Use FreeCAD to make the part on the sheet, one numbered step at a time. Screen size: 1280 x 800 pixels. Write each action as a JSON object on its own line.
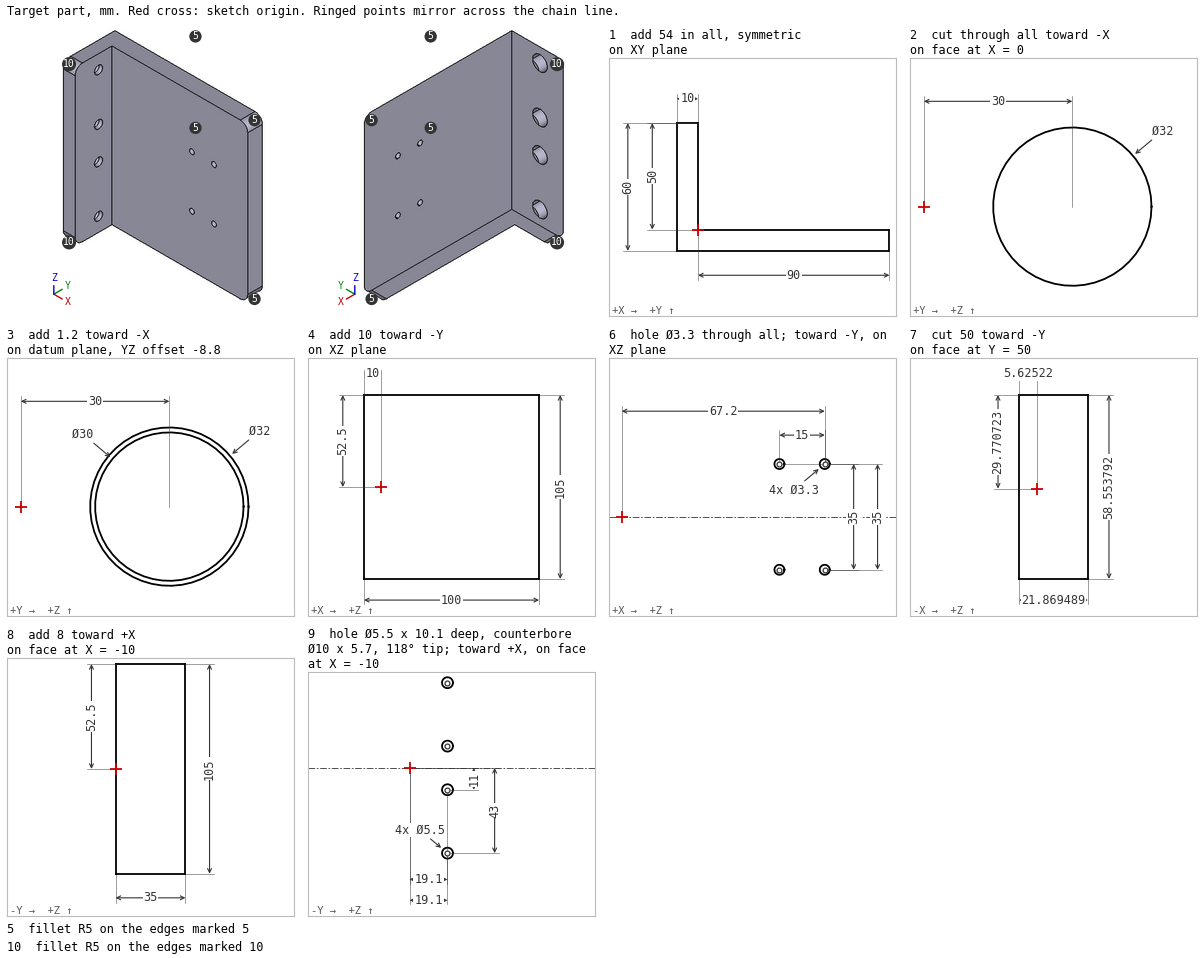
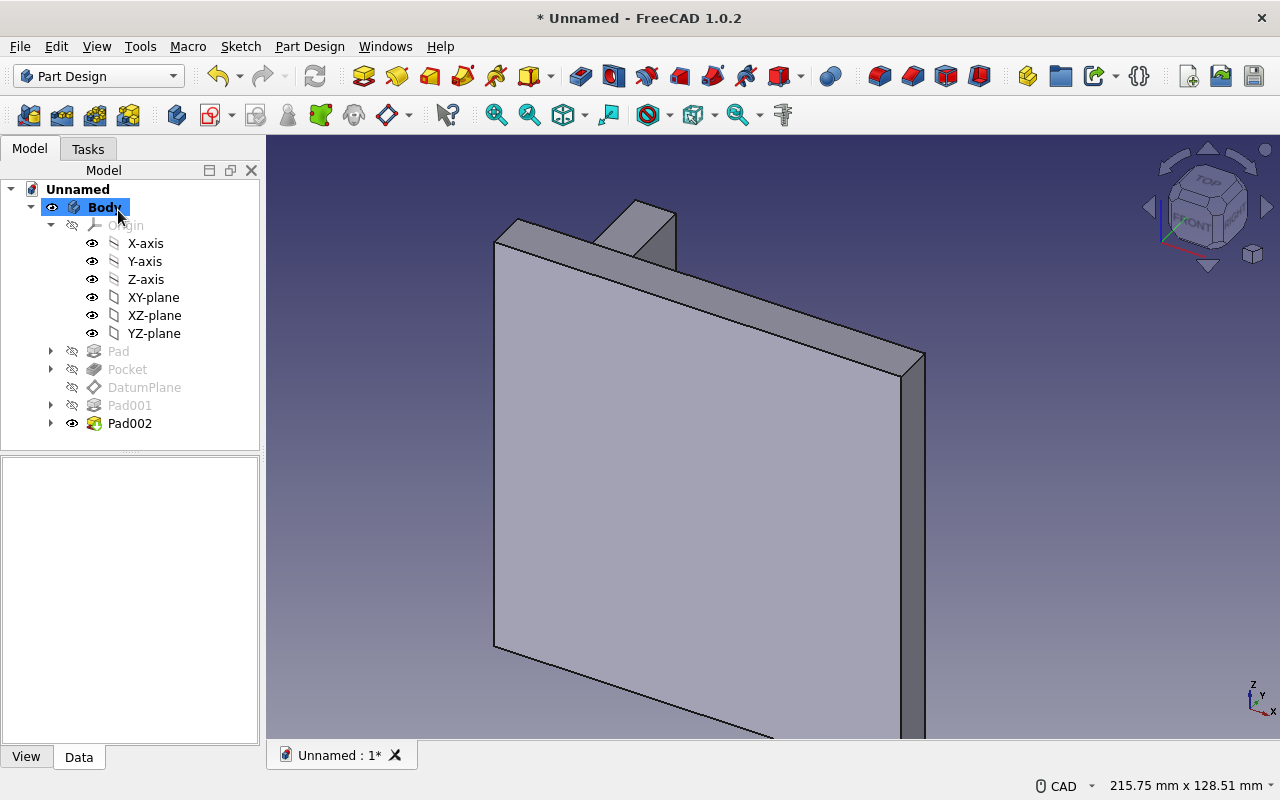
{"action": "left_click", "coordinate": [497, 116]}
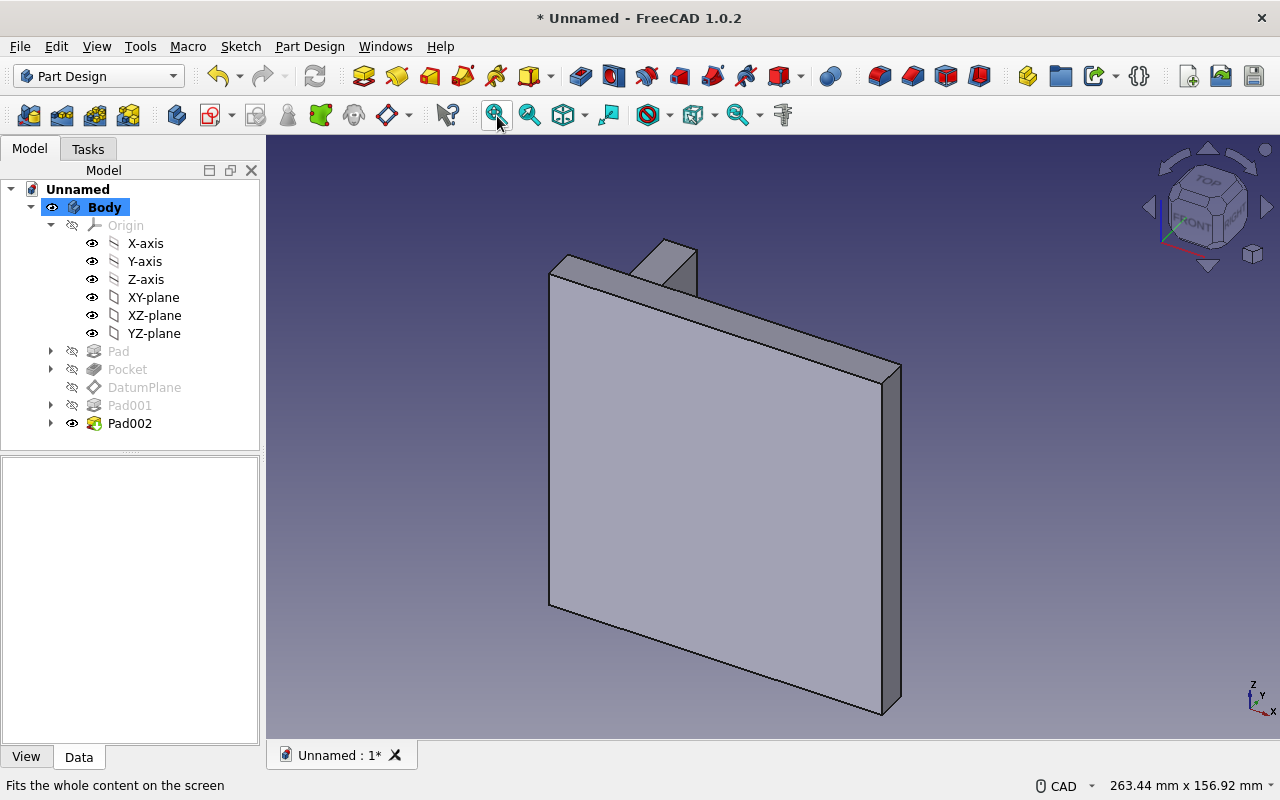
{"action": "left_click", "coordinate": [892, 373]}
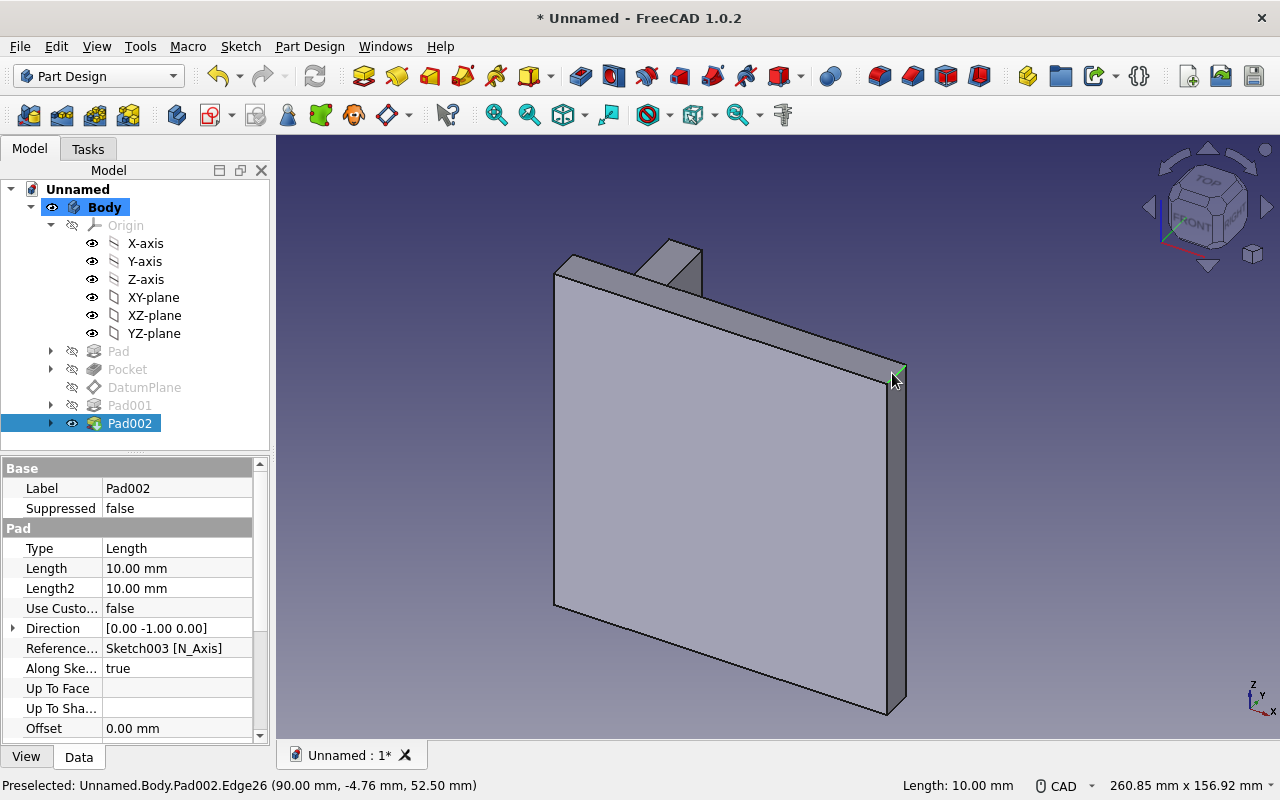
{"action": "key", "text": "0"}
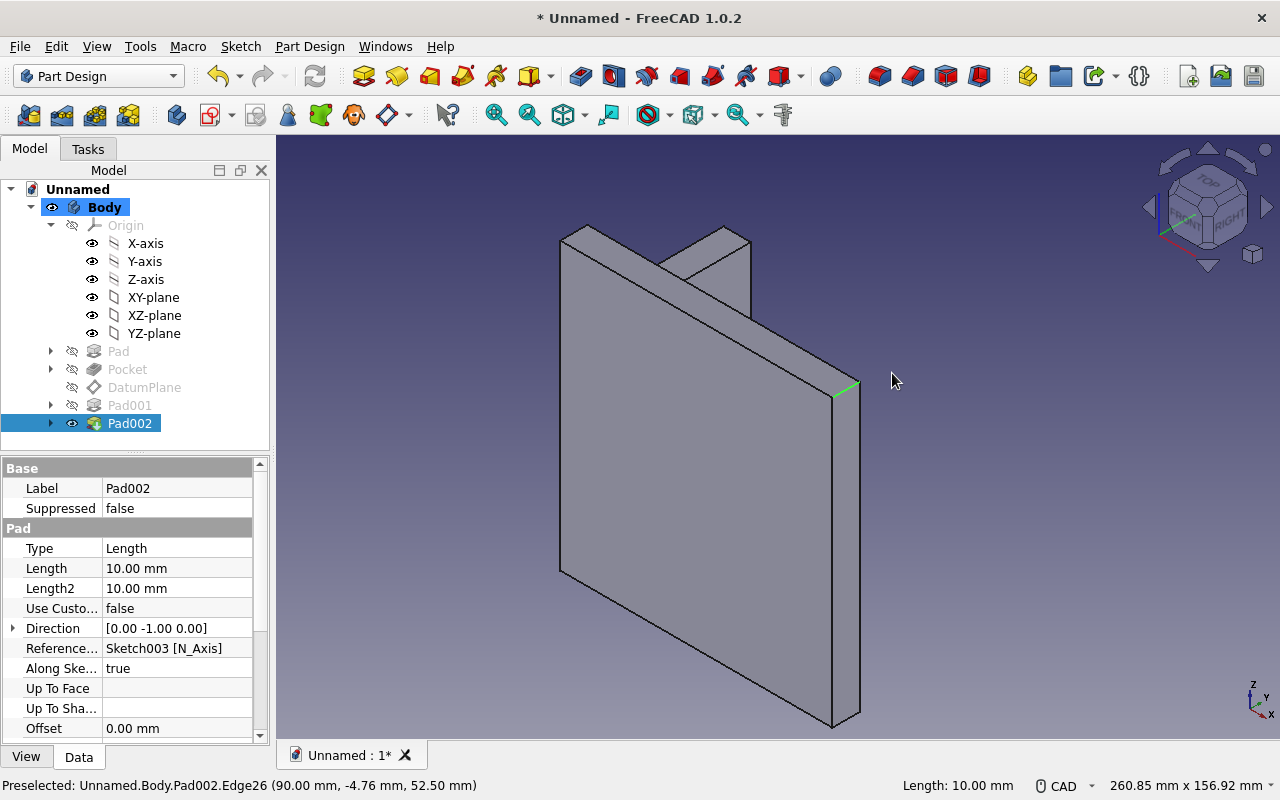
{"action": "key", "text": "2"}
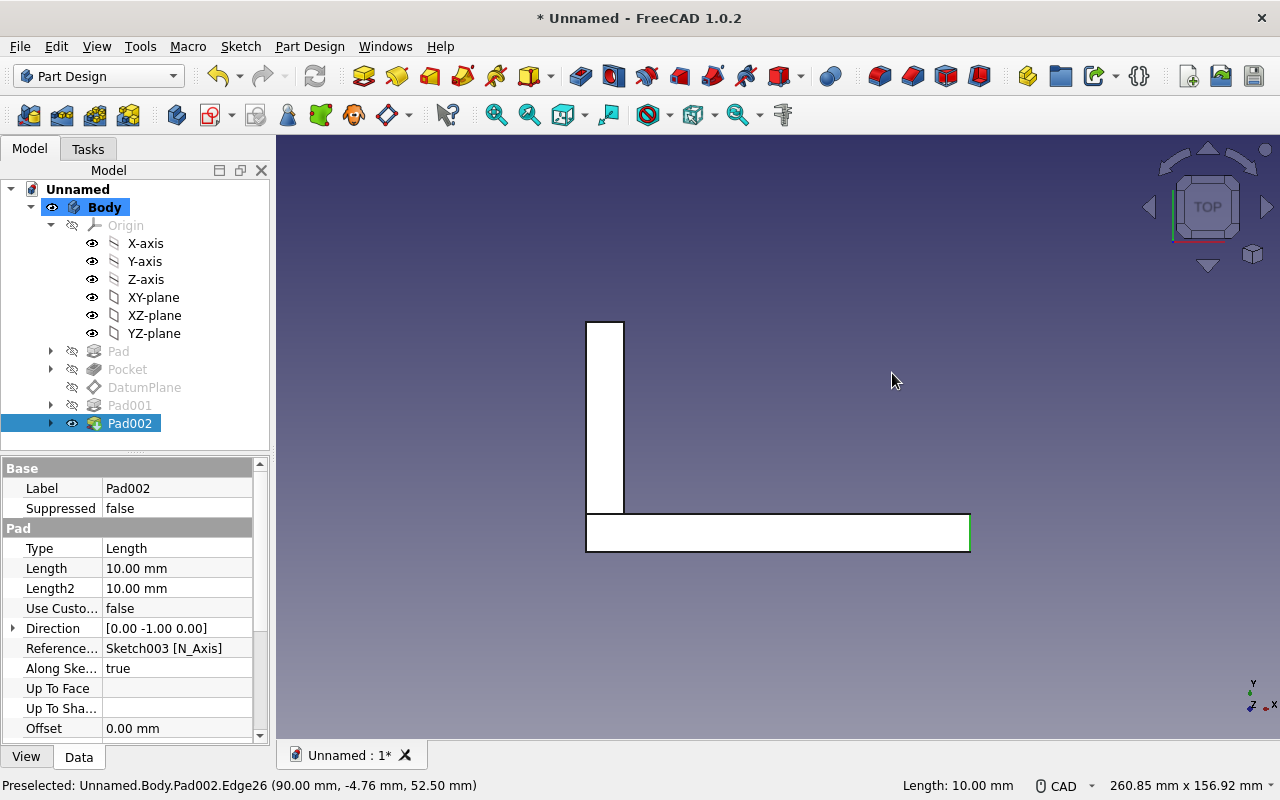
{"action": "left_click", "coordinate": [497, 116]}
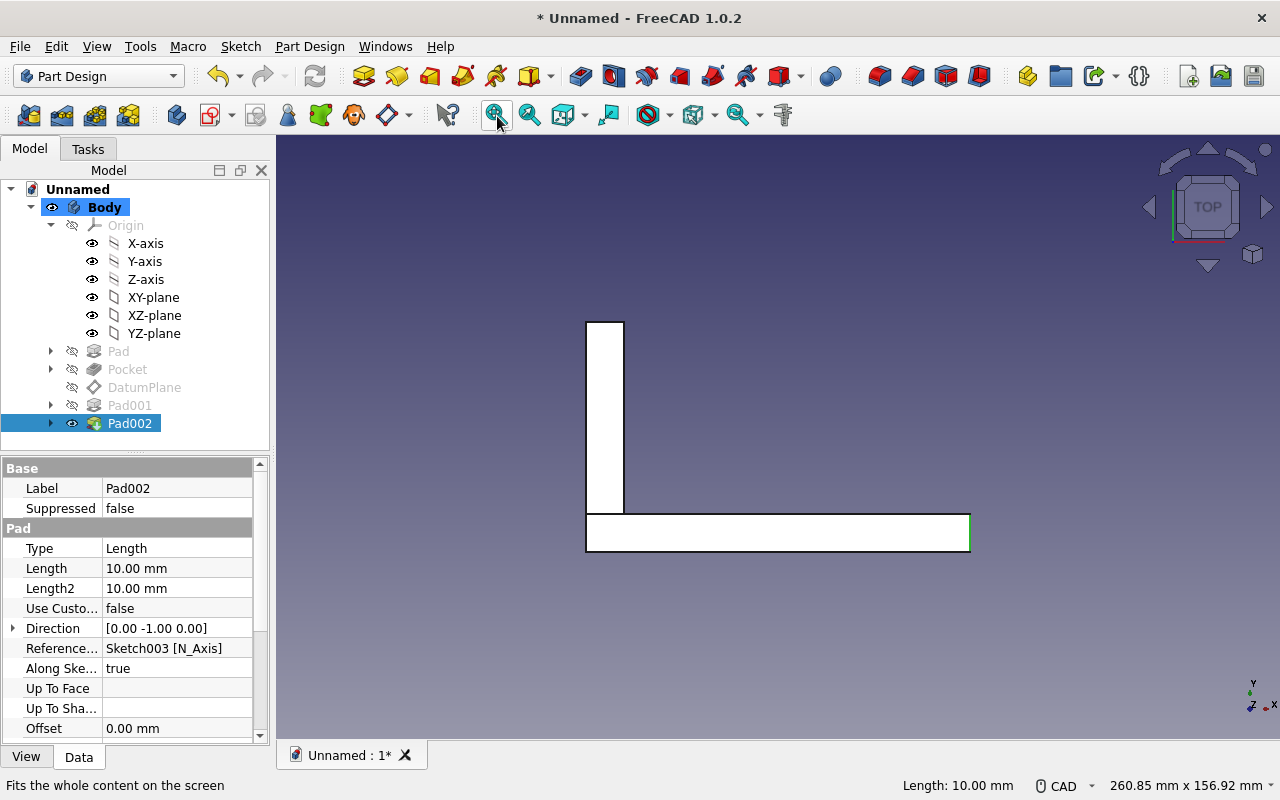
{"action": "left_click", "coordinate": [605, 321], "text": "ctrl"}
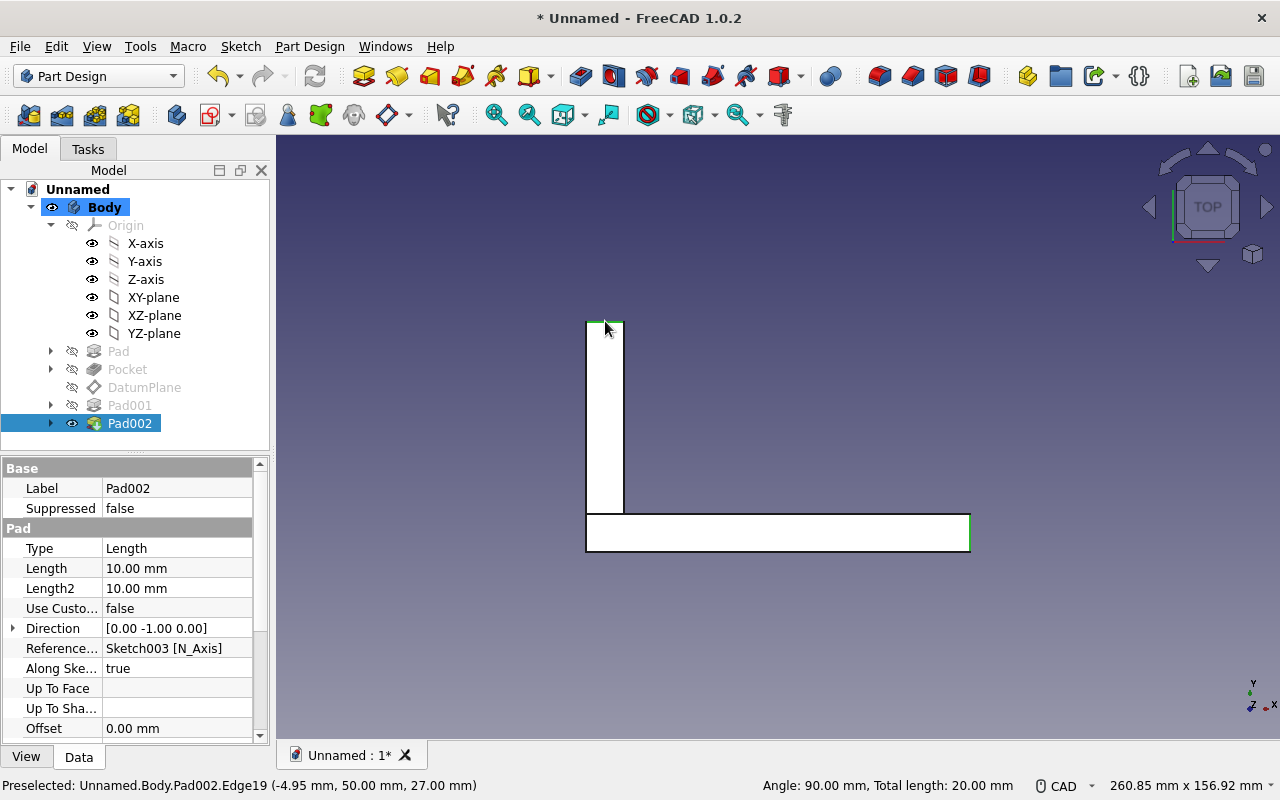
{"action": "key", "text": "1"}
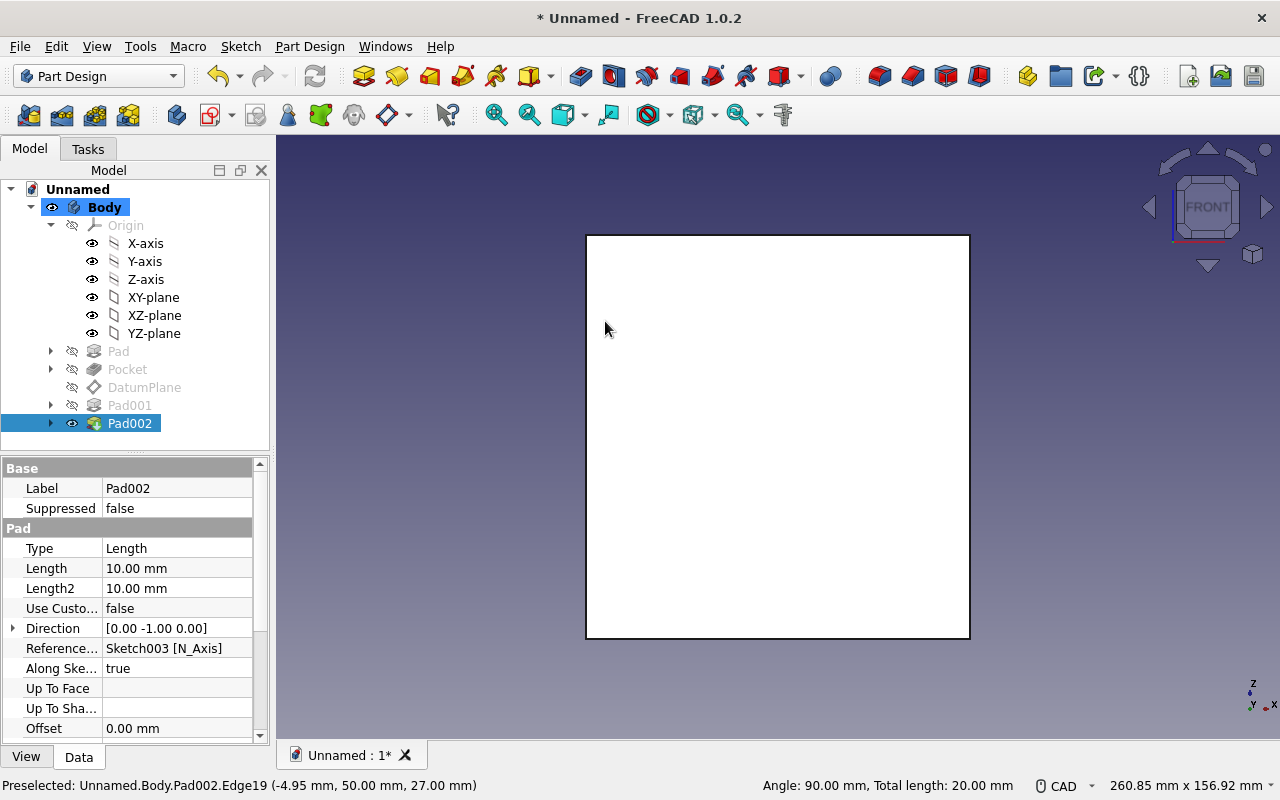
{"action": "key", "text": "3"}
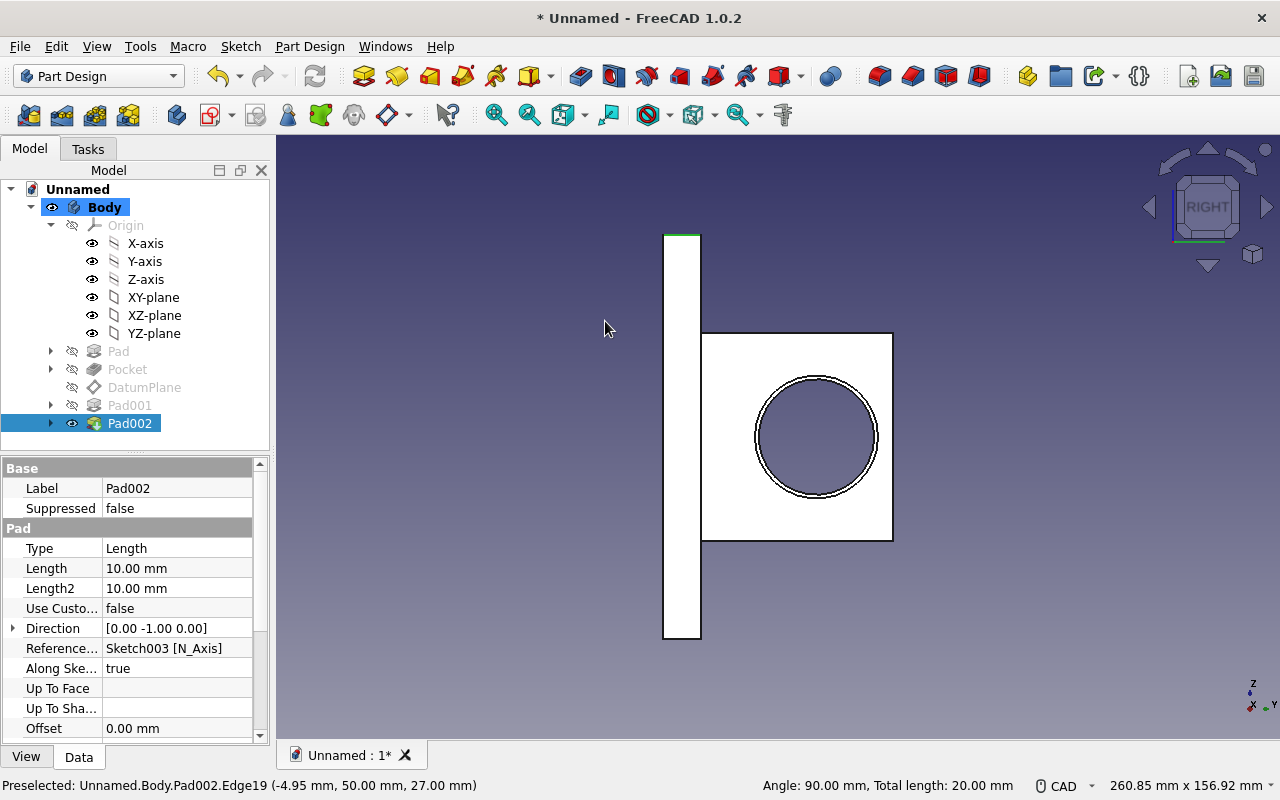
{"action": "left_click", "coordinate": [682, 638], "text": "ctrl"}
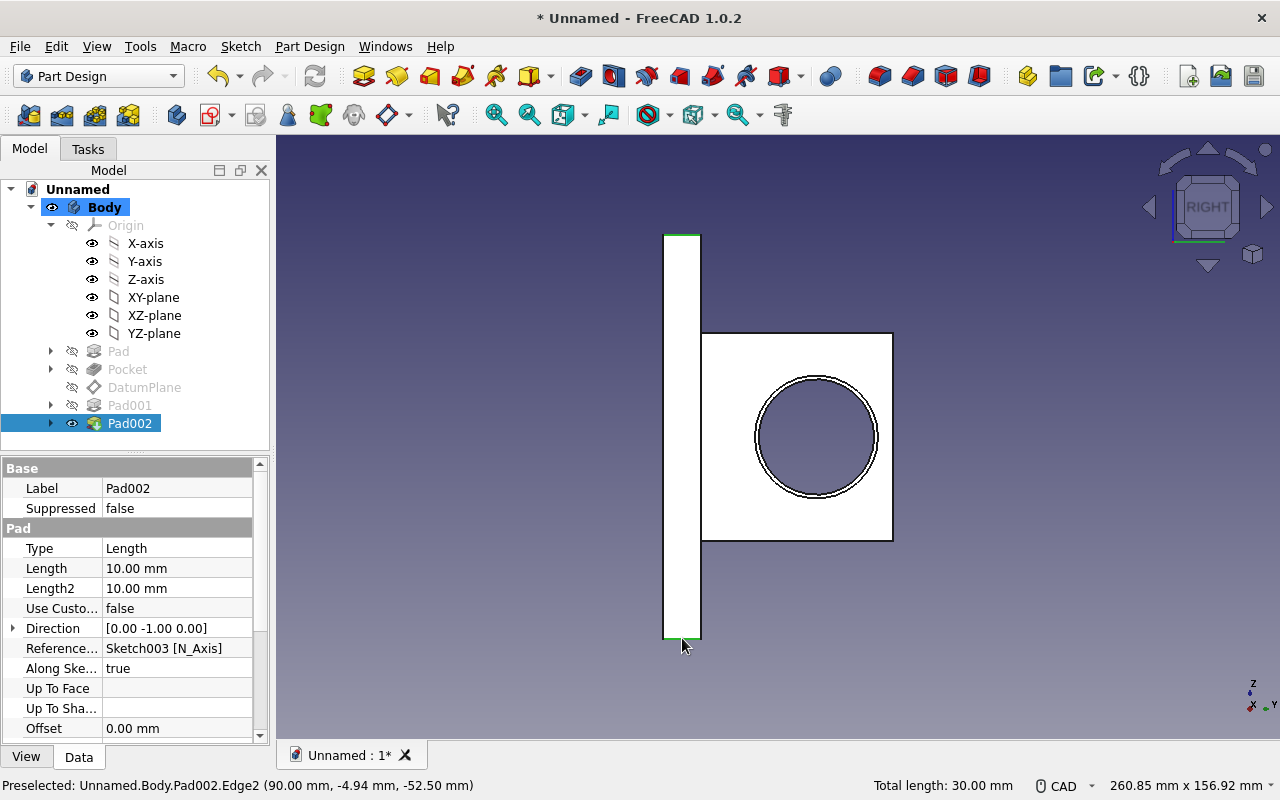
{"action": "key", "text": "5"}